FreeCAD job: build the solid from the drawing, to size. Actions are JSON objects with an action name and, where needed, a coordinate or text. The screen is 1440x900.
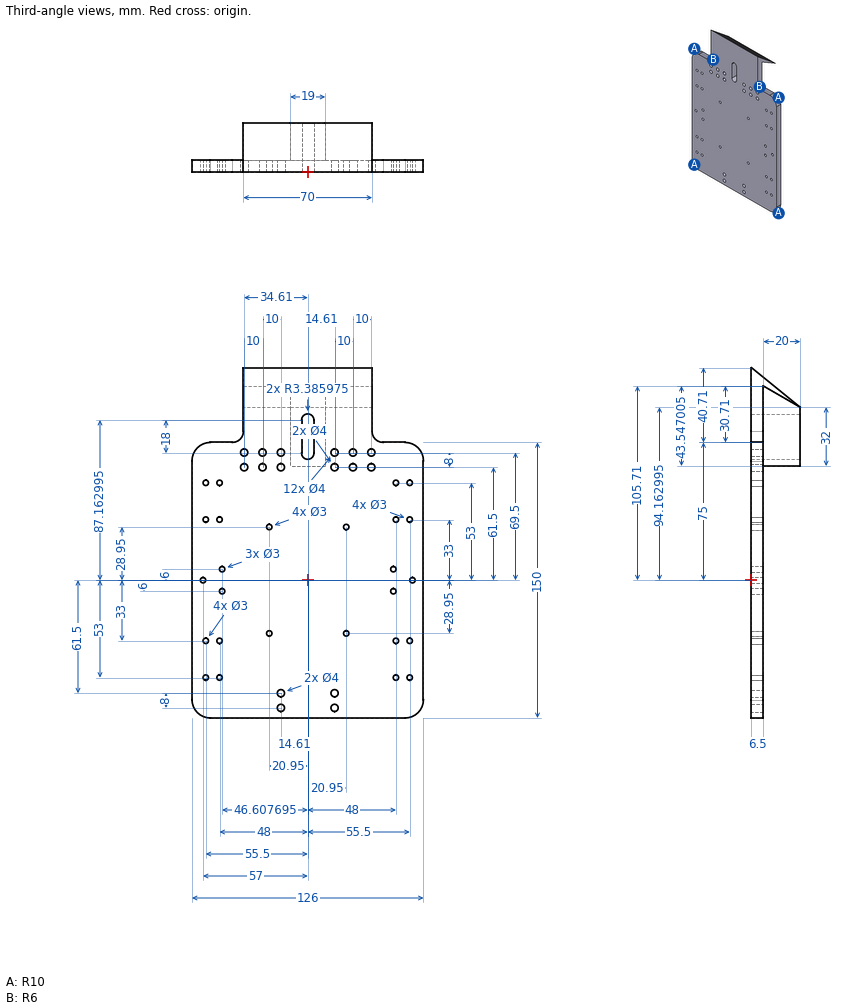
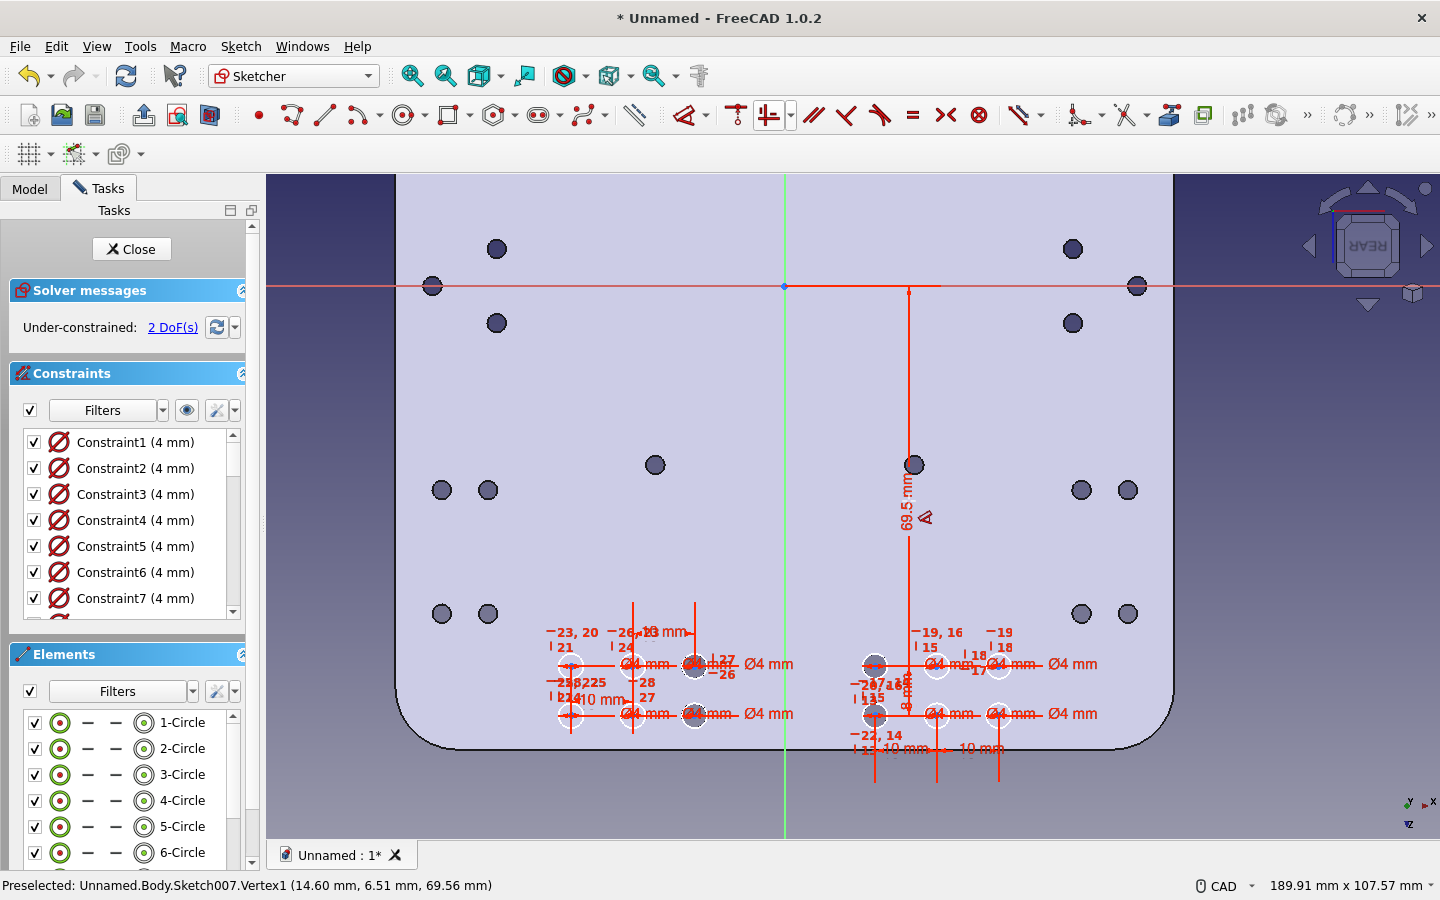
{"action": "left_click", "coordinate": [875, 716]}
{"action": "left_click", "coordinate": [830, 252]}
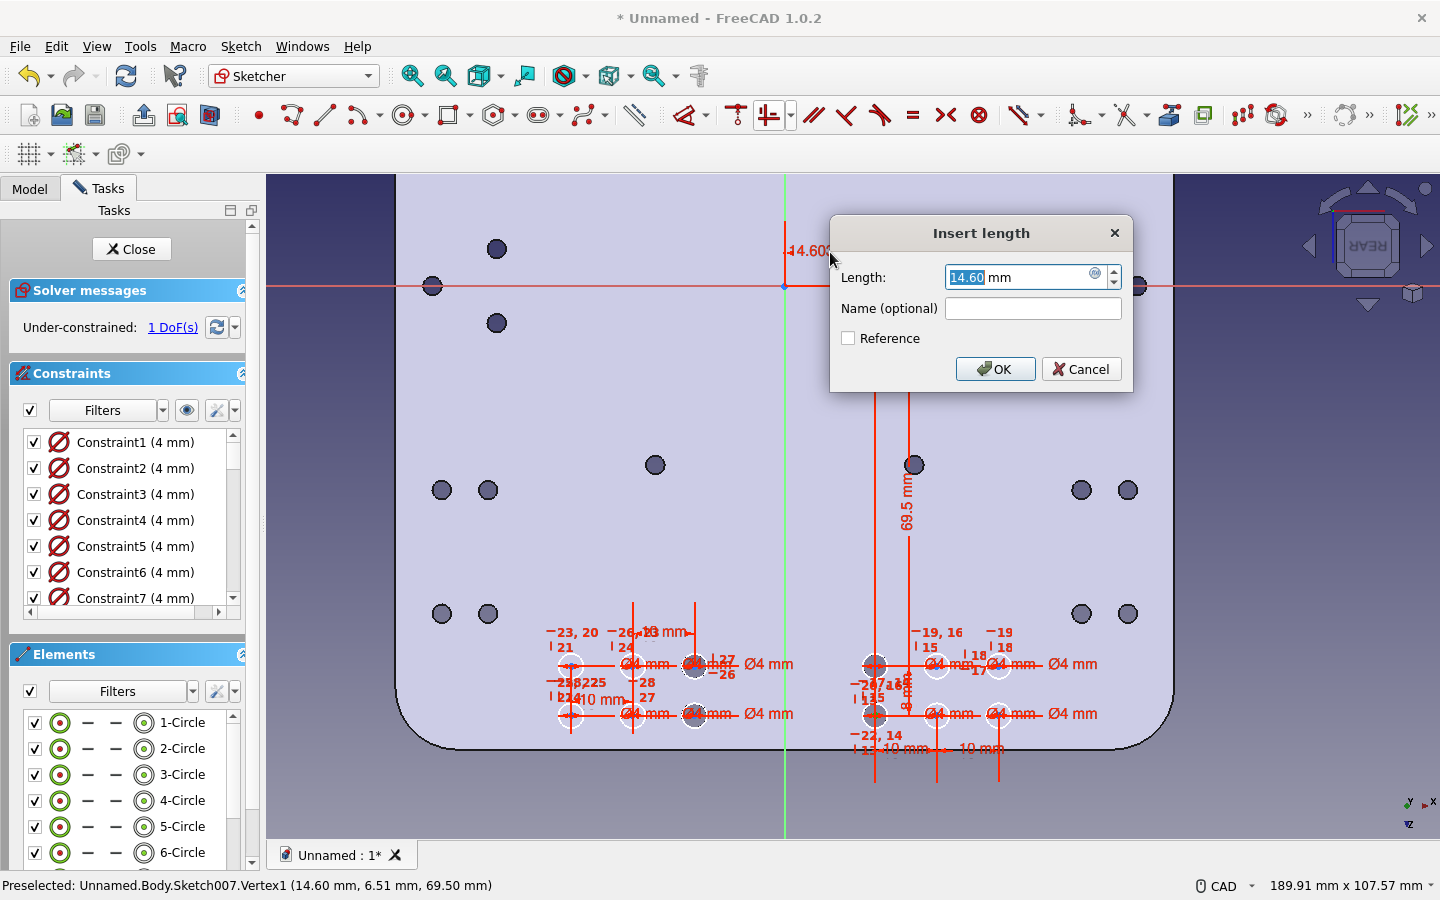
{"action": "type", "text": "14.61"}
{"action": "key", "text": "Return"}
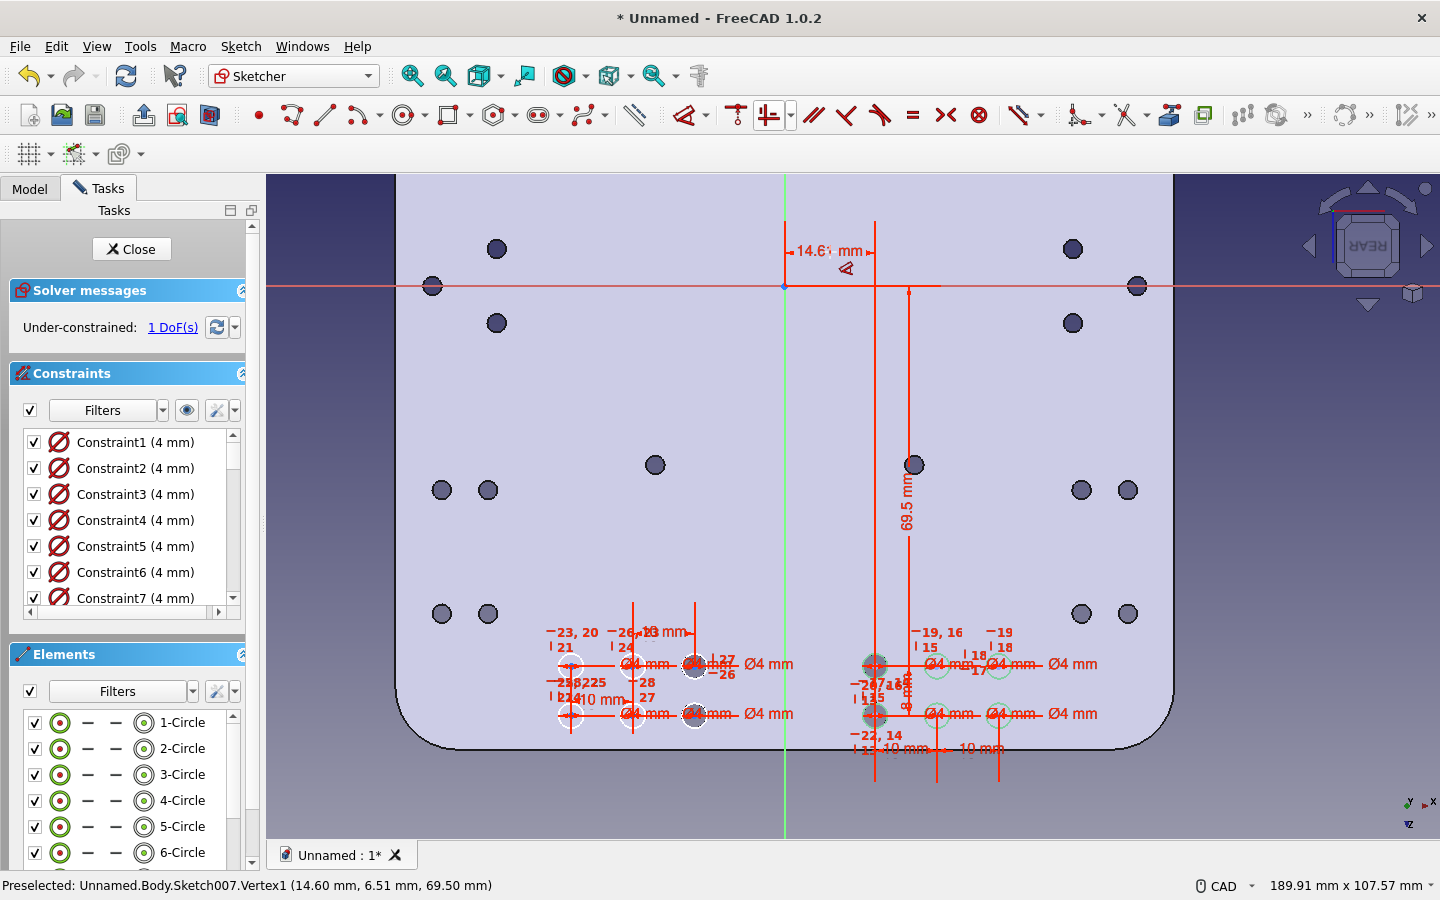
{"action": "left_click", "coordinate": [571, 666]}
{"action": "left_click", "coordinate": [678, 252]}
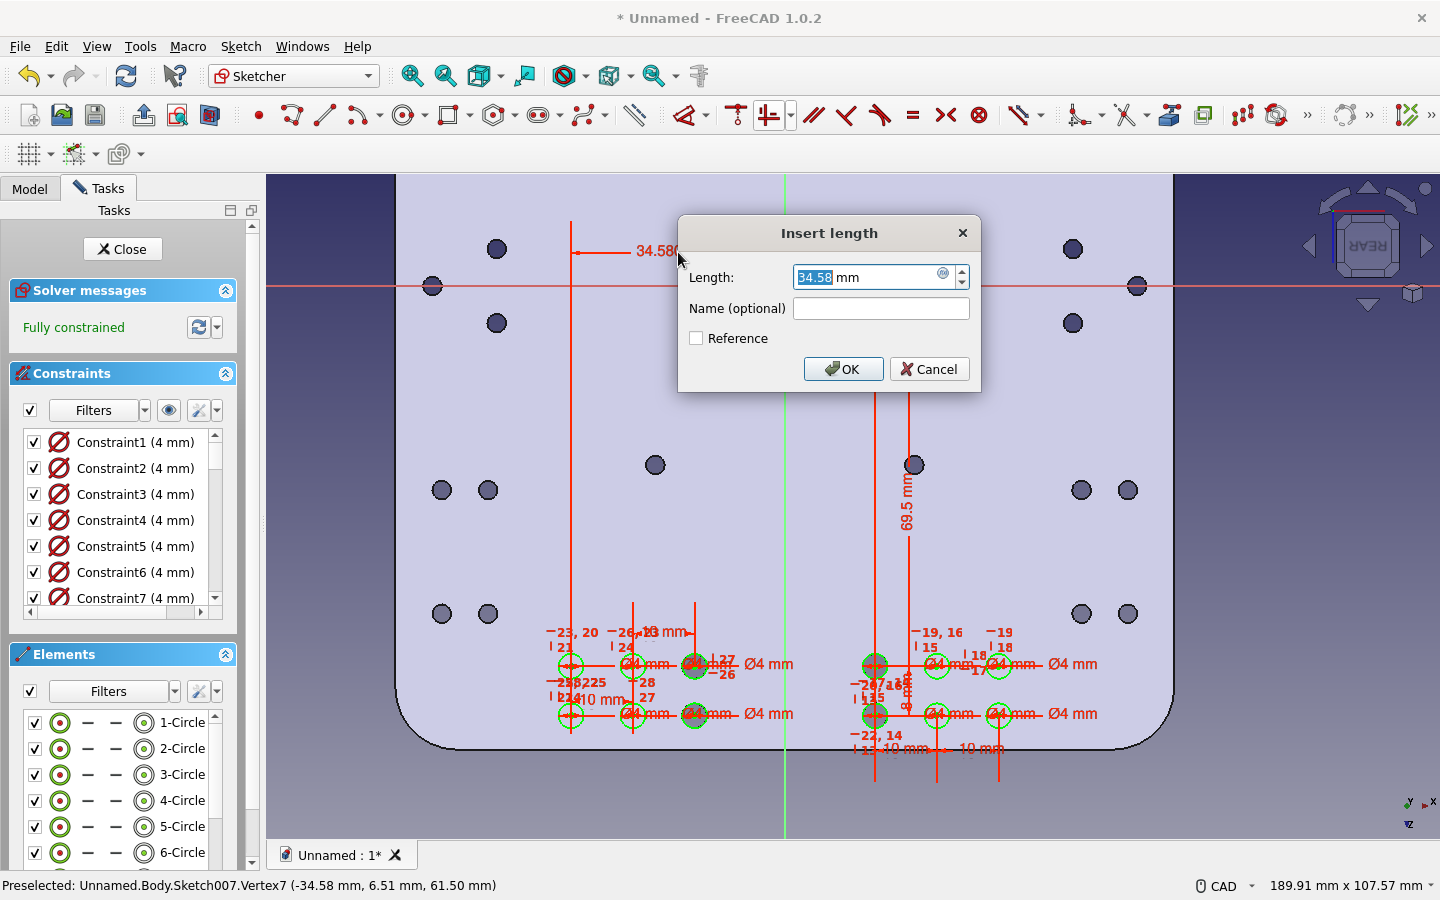
{"action": "type", "text": "34.61"}
{"action": "key", "text": "Return"}
{"action": "key", "text": "Escape"}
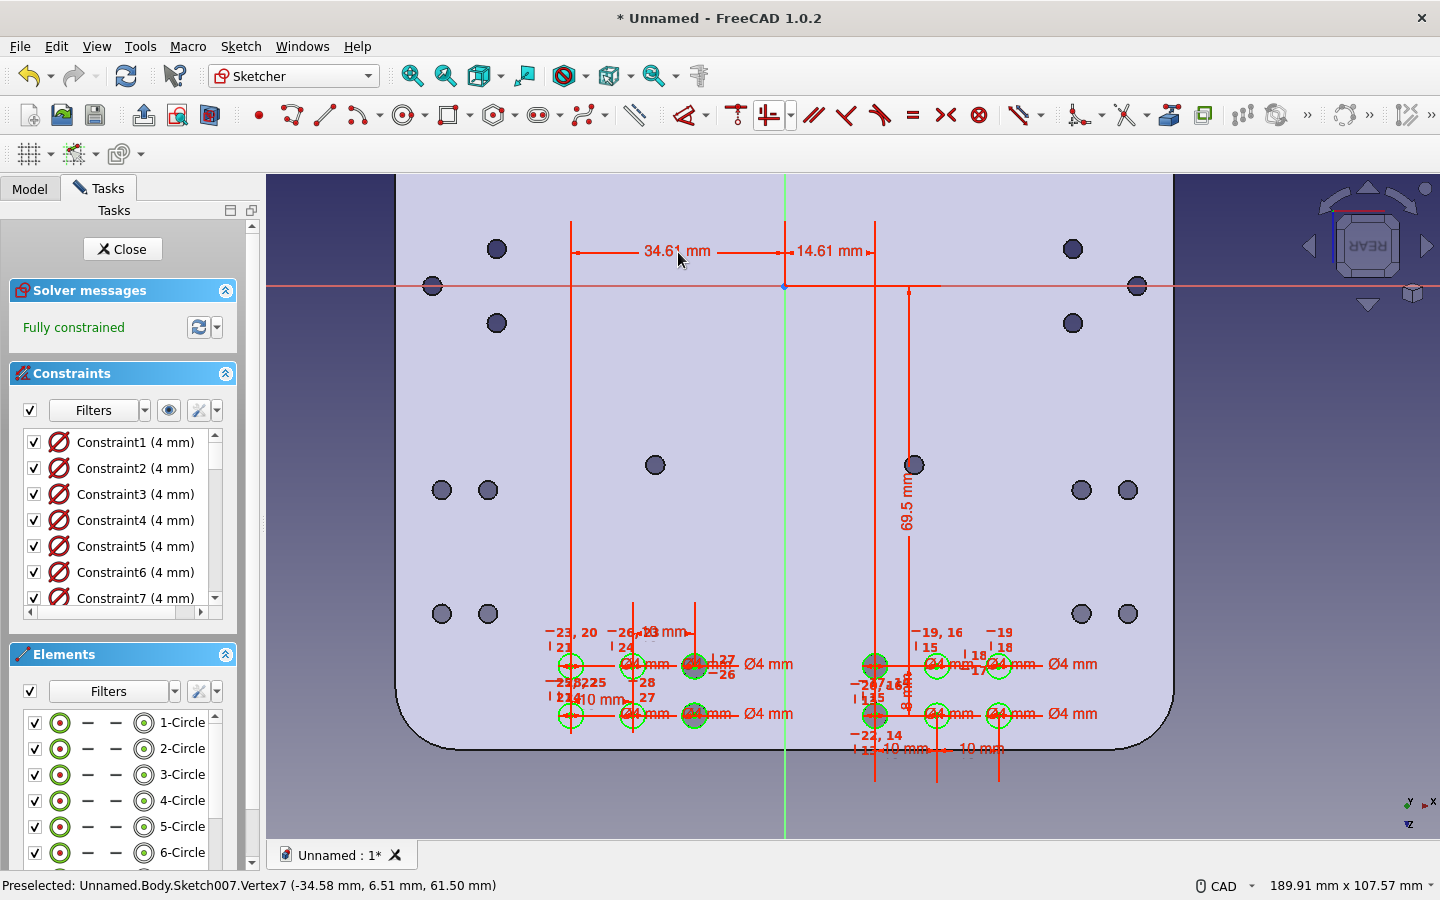
{"action": "left_click", "coordinate": [123, 249]}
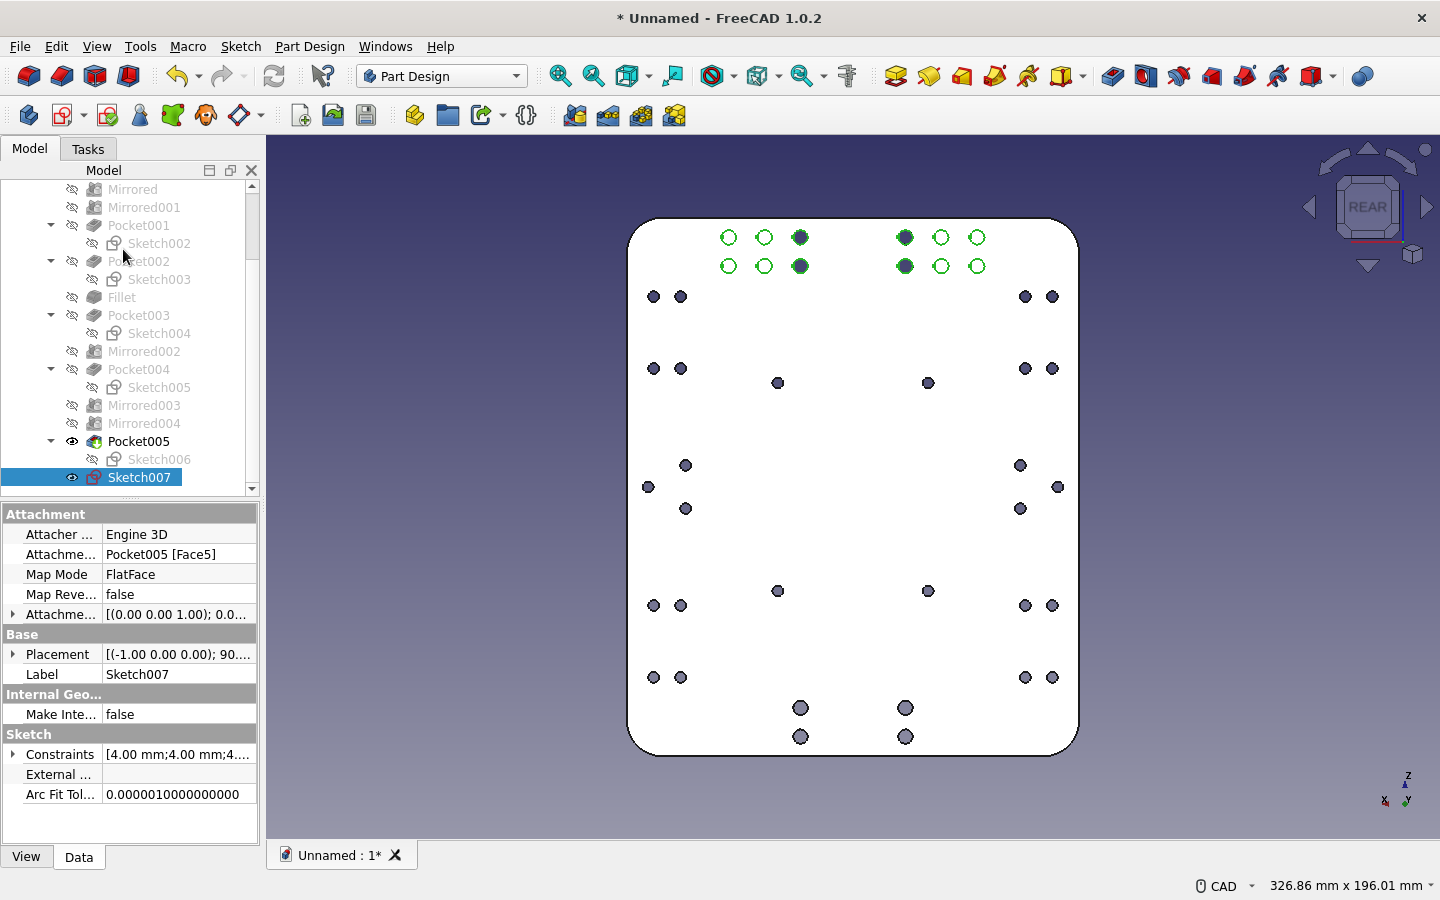
{"action": "left_click", "coordinate": [1113, 76]}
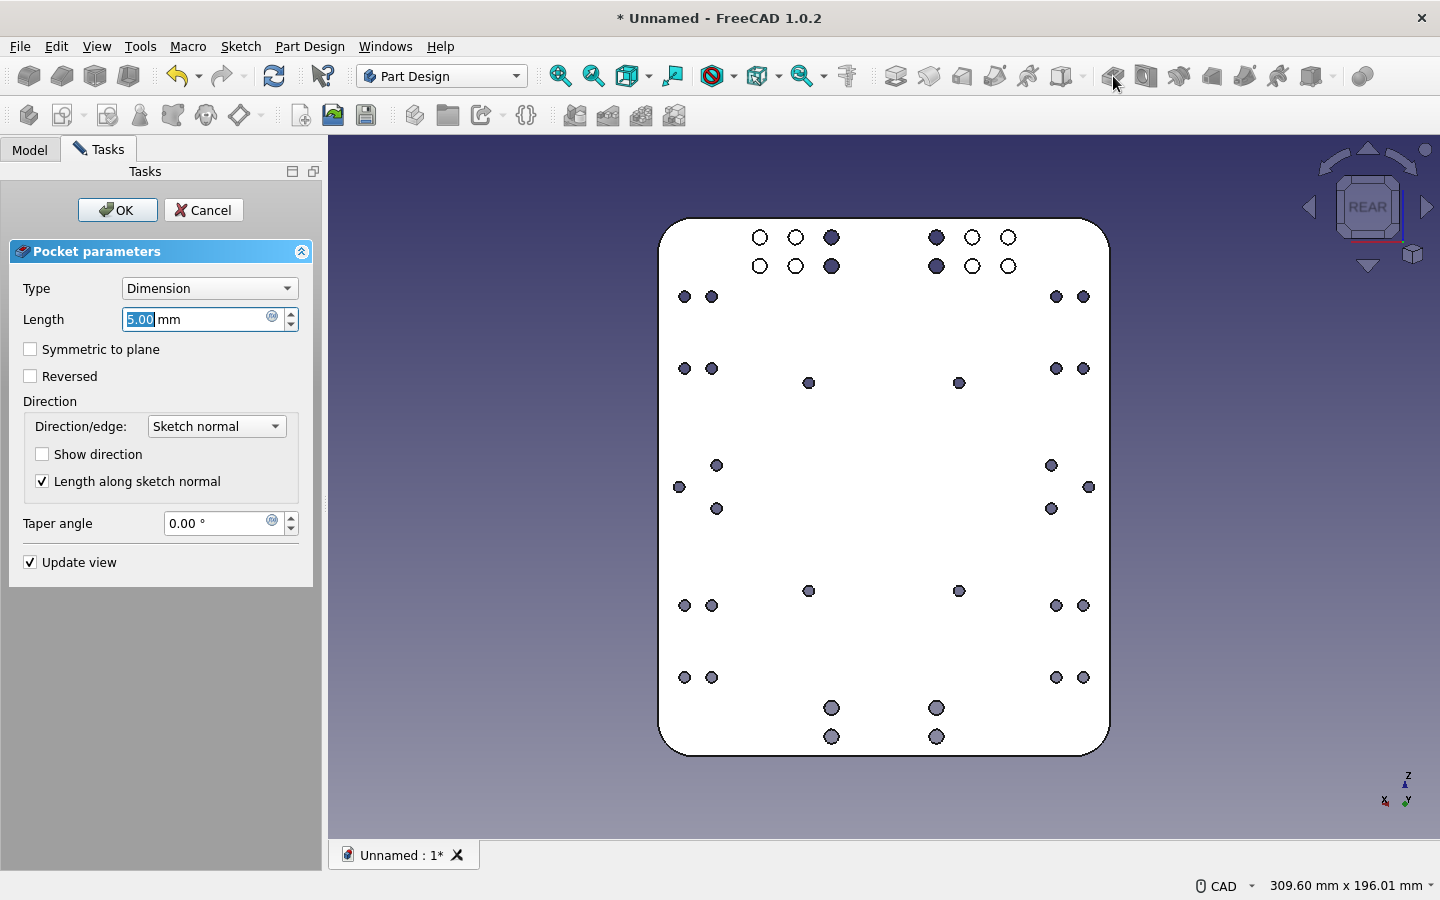
{"action": "left_click", "coordinate": [210, 288]}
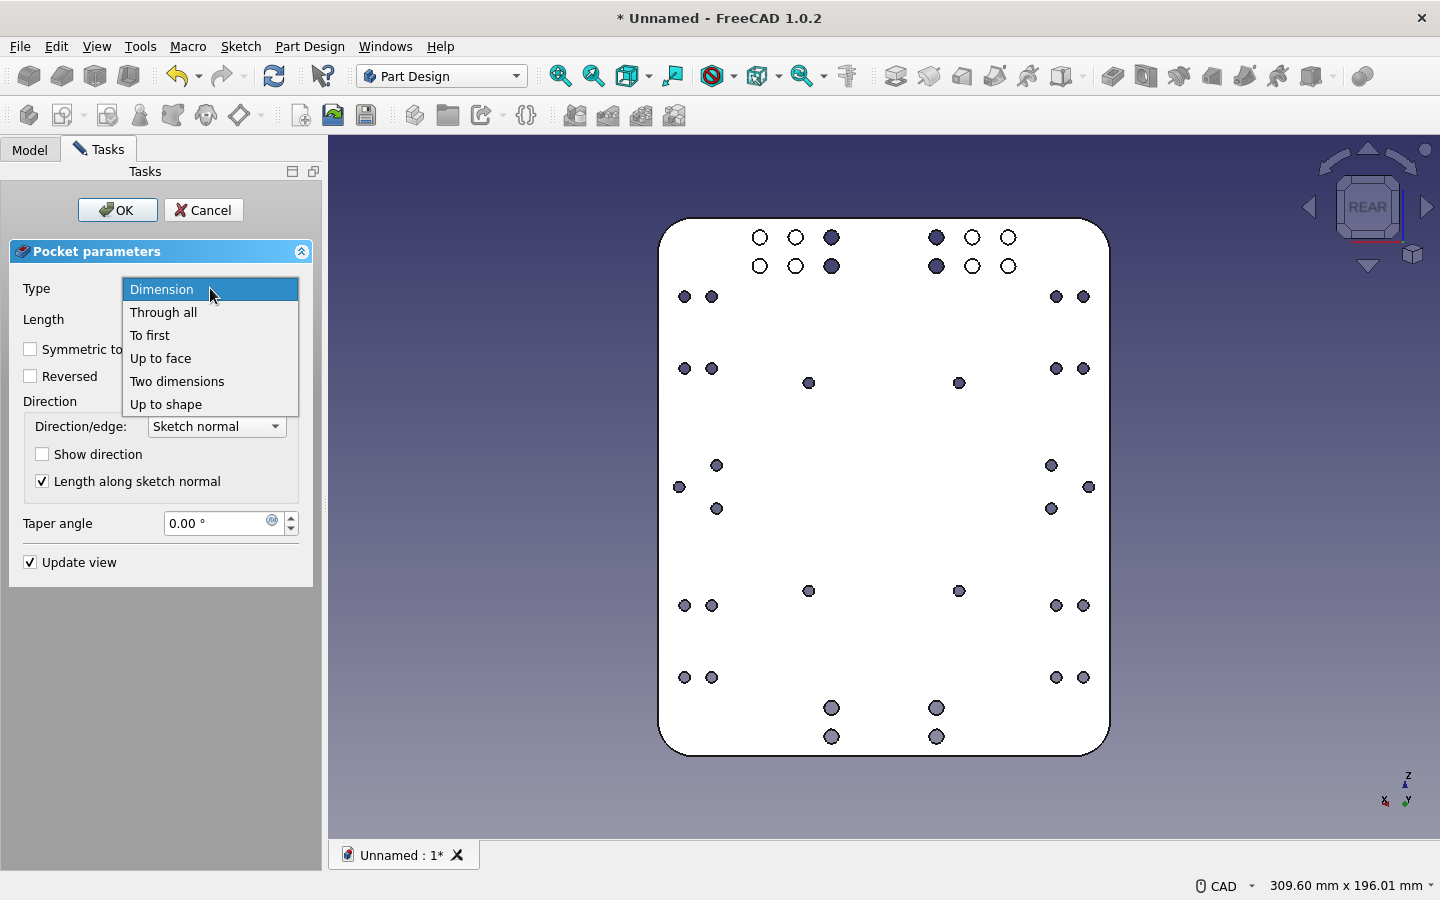
{"action": "left_click", "coordinate": [208, 312]}